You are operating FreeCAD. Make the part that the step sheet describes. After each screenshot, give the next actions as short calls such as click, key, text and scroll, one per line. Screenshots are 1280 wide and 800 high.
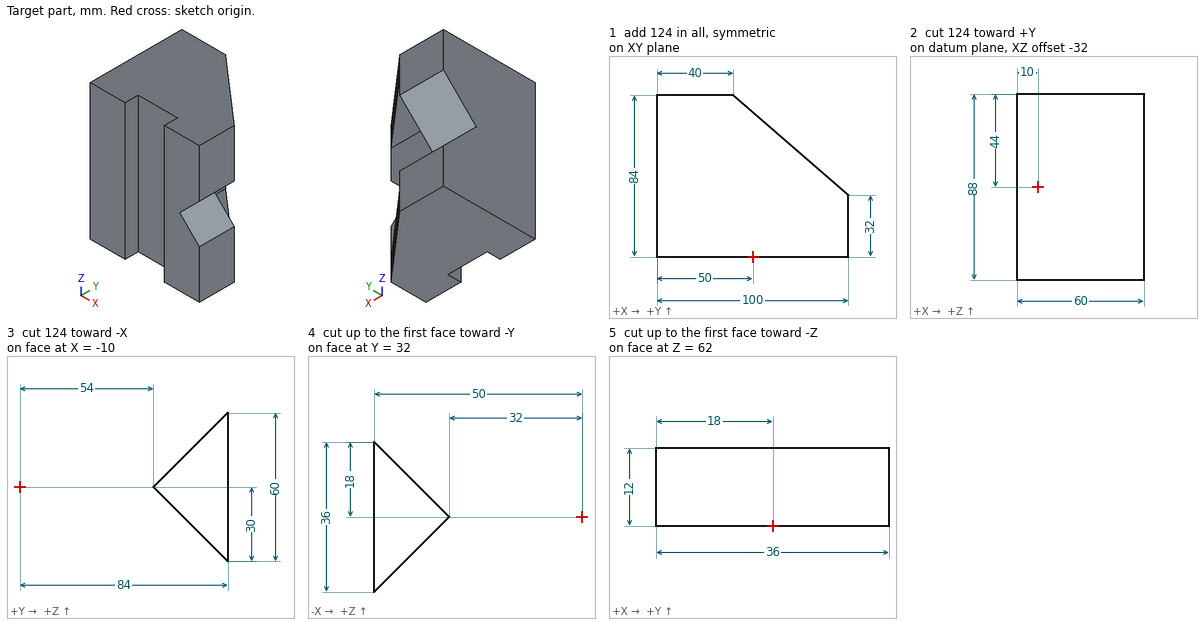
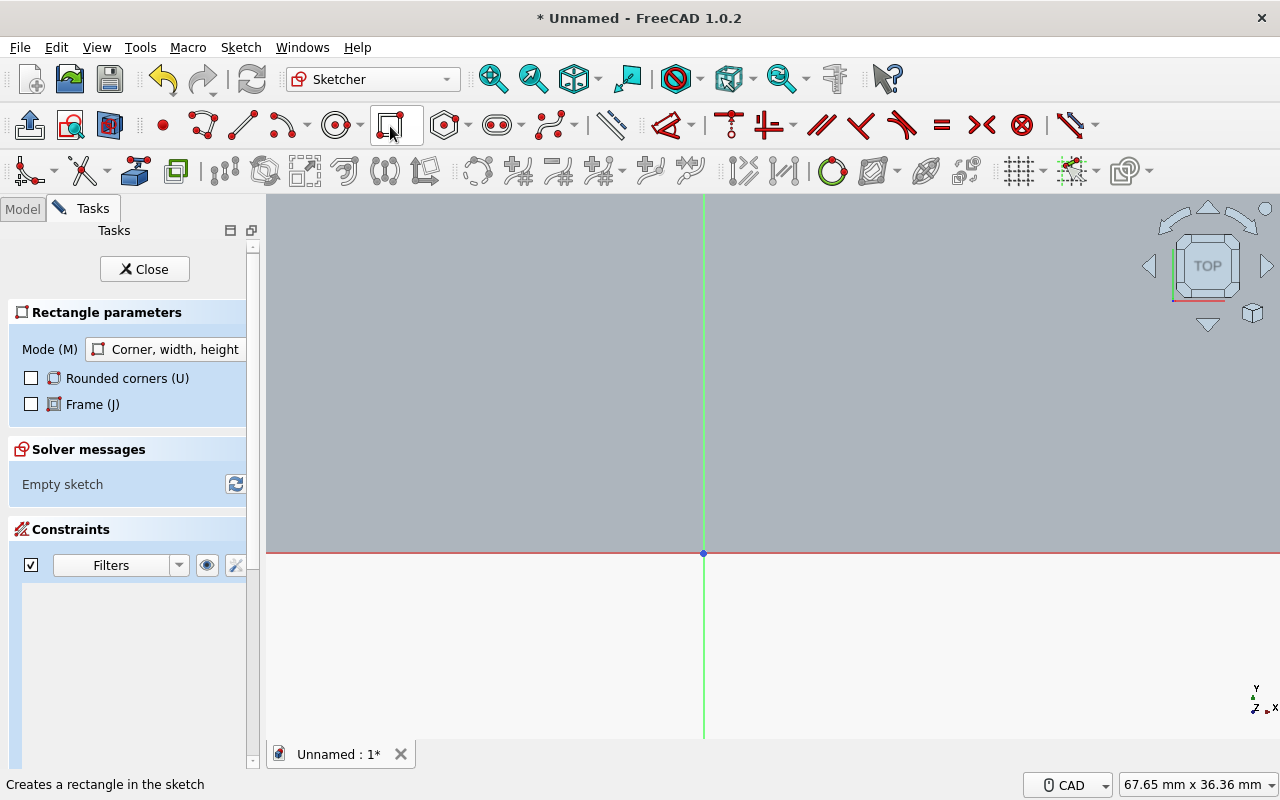
click(434, 374)
click(974, 553)
key(Escape)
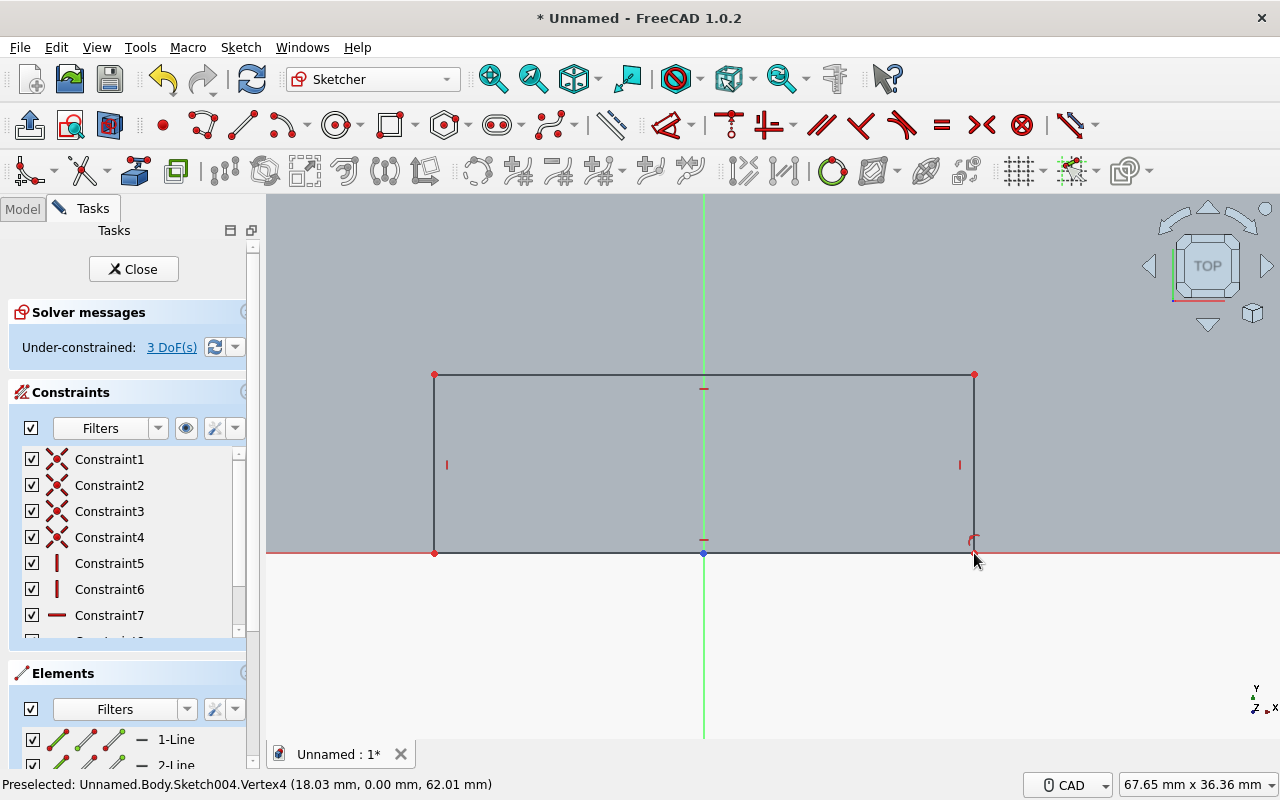
click(666, 126)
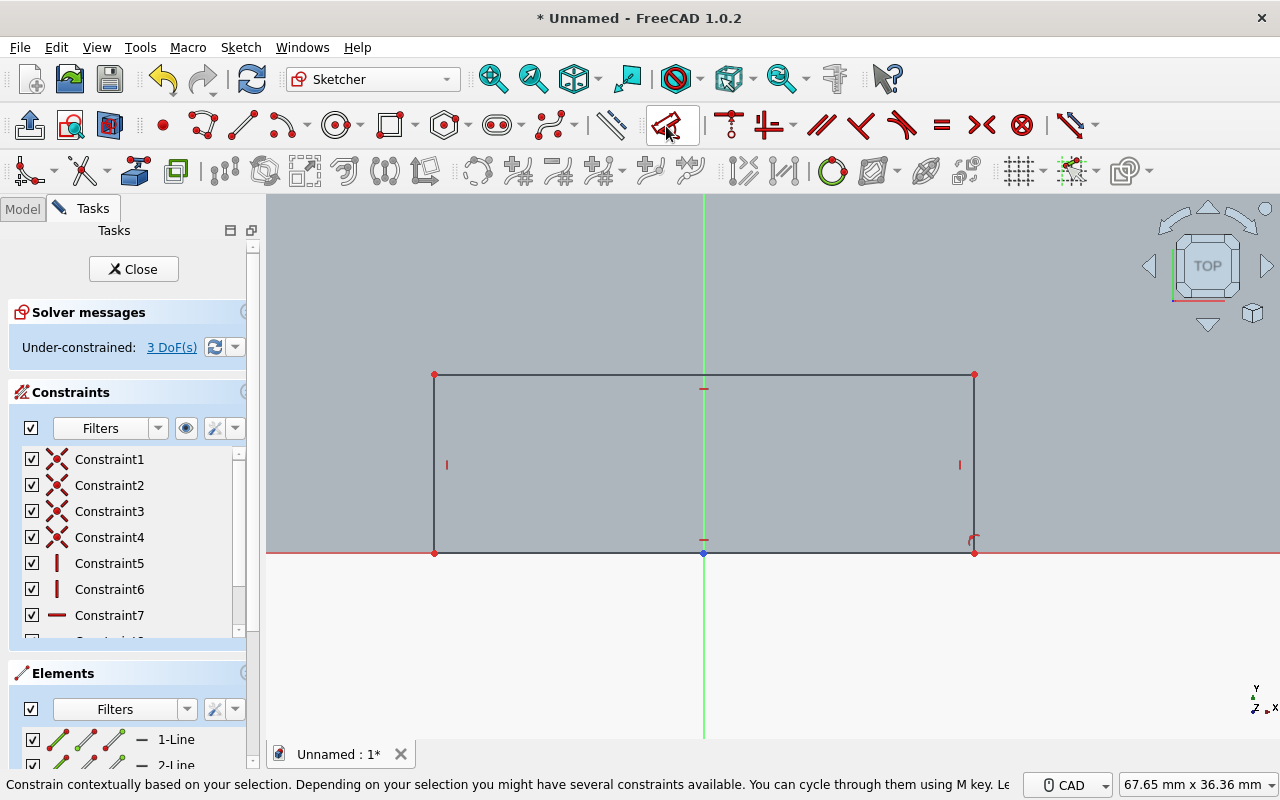
click(434, 429)
click(400, 464)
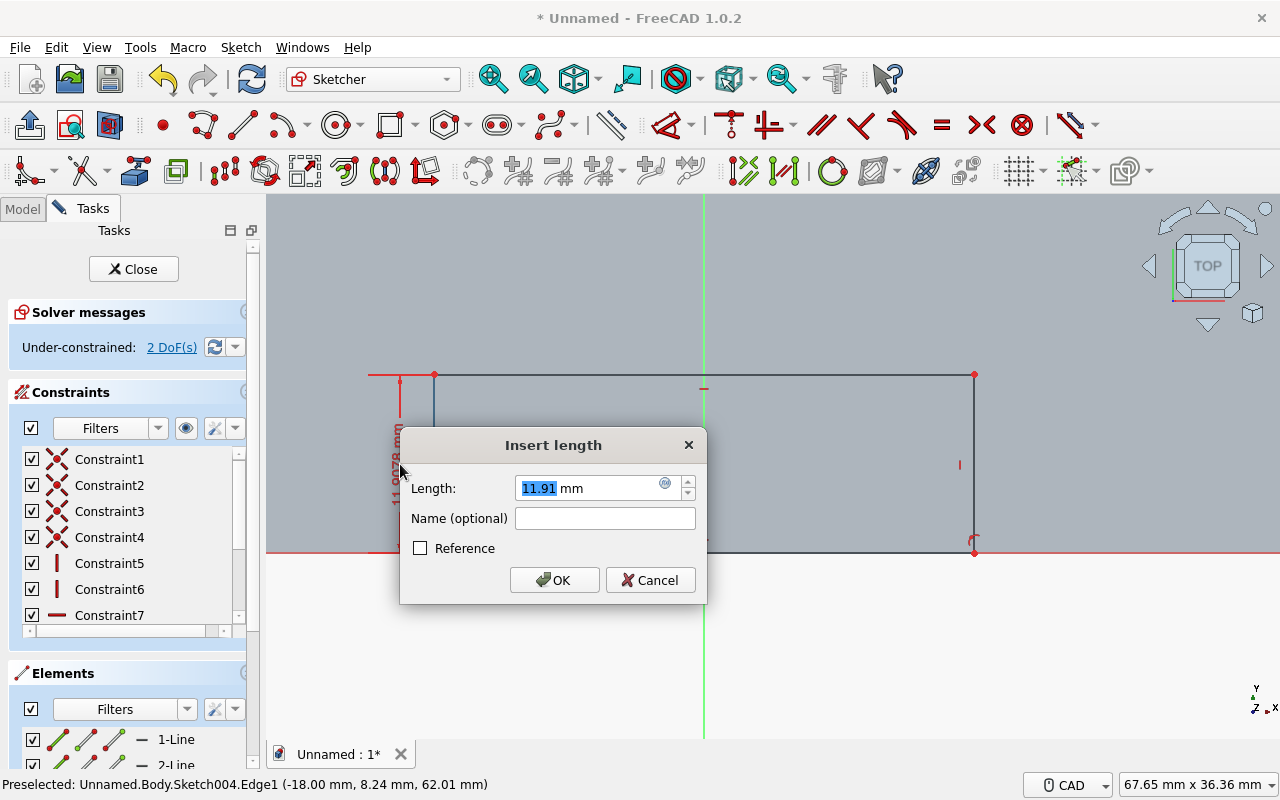
text(12)
key(Return)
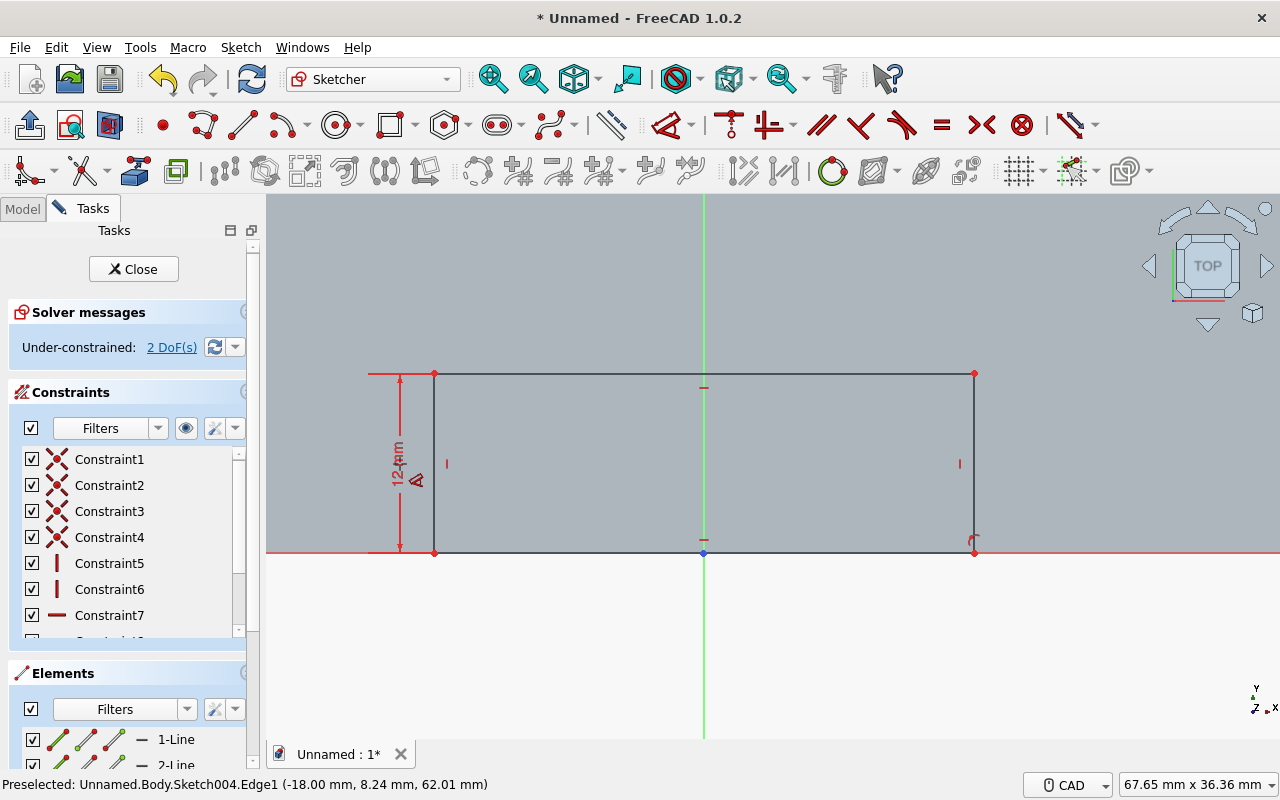
click(596, 553)
click(580, 587)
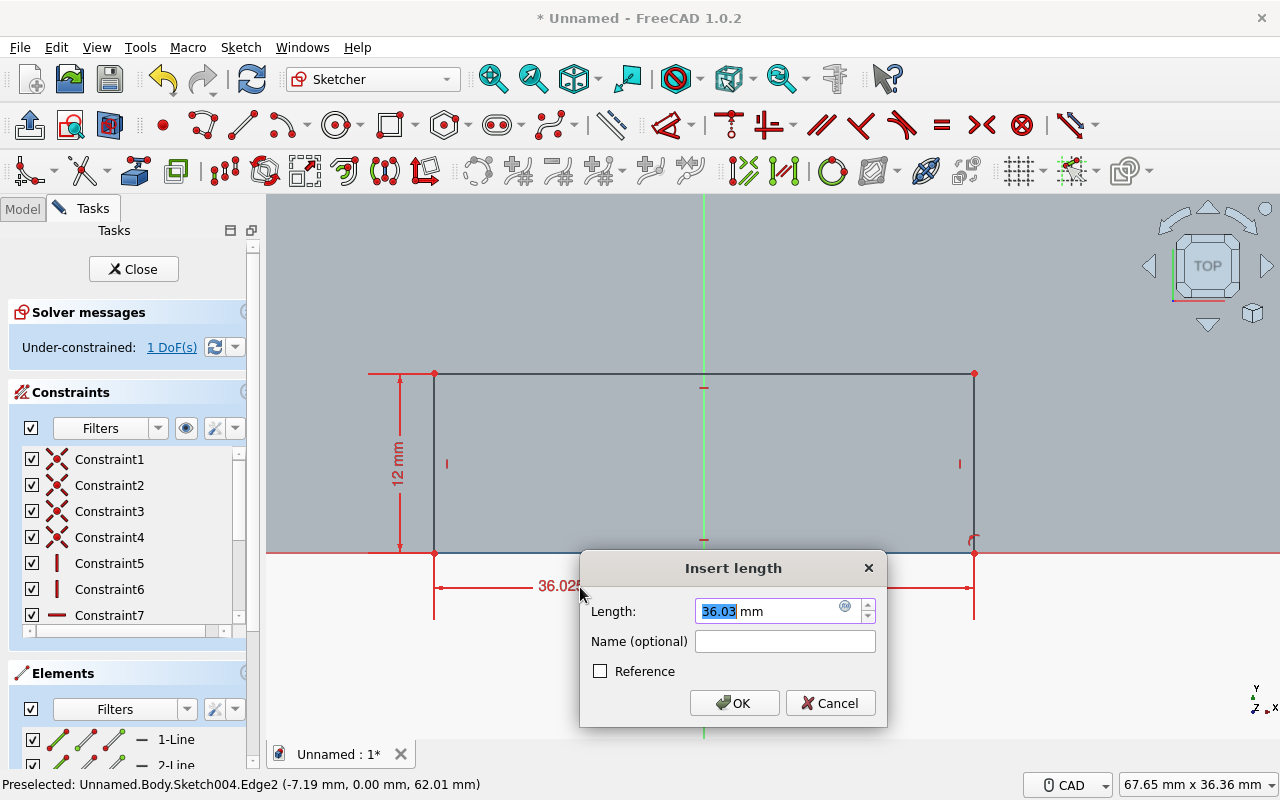
text(36)
key(Return)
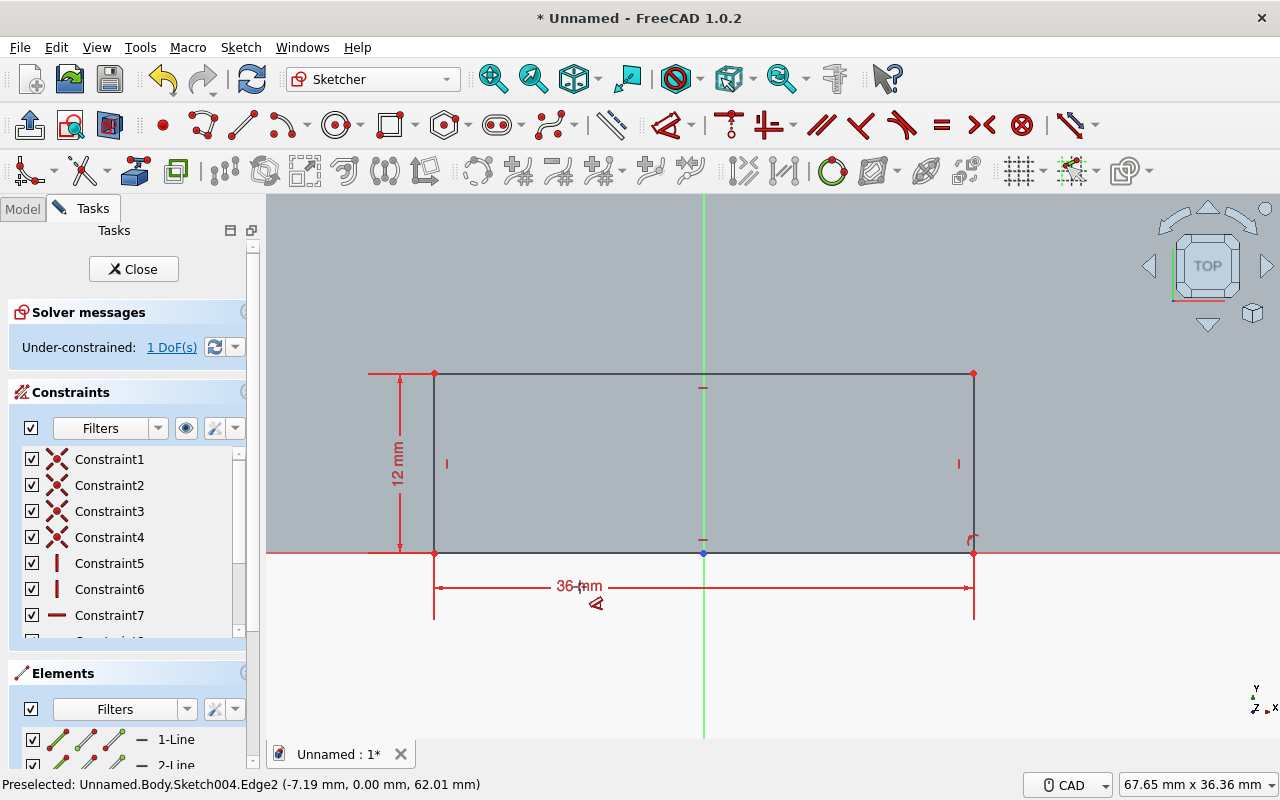
click(434, 374)
click(507, 587)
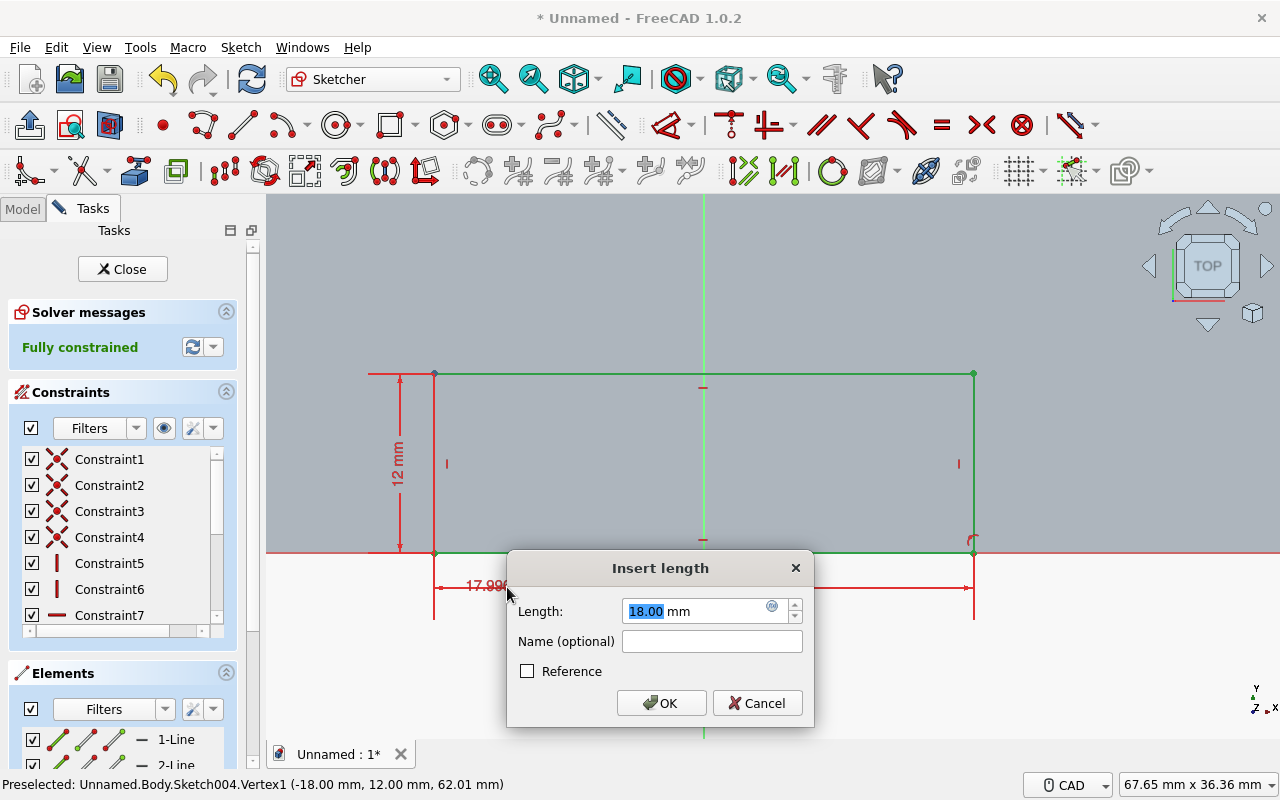
text(18)
key(Return)
key(Escape)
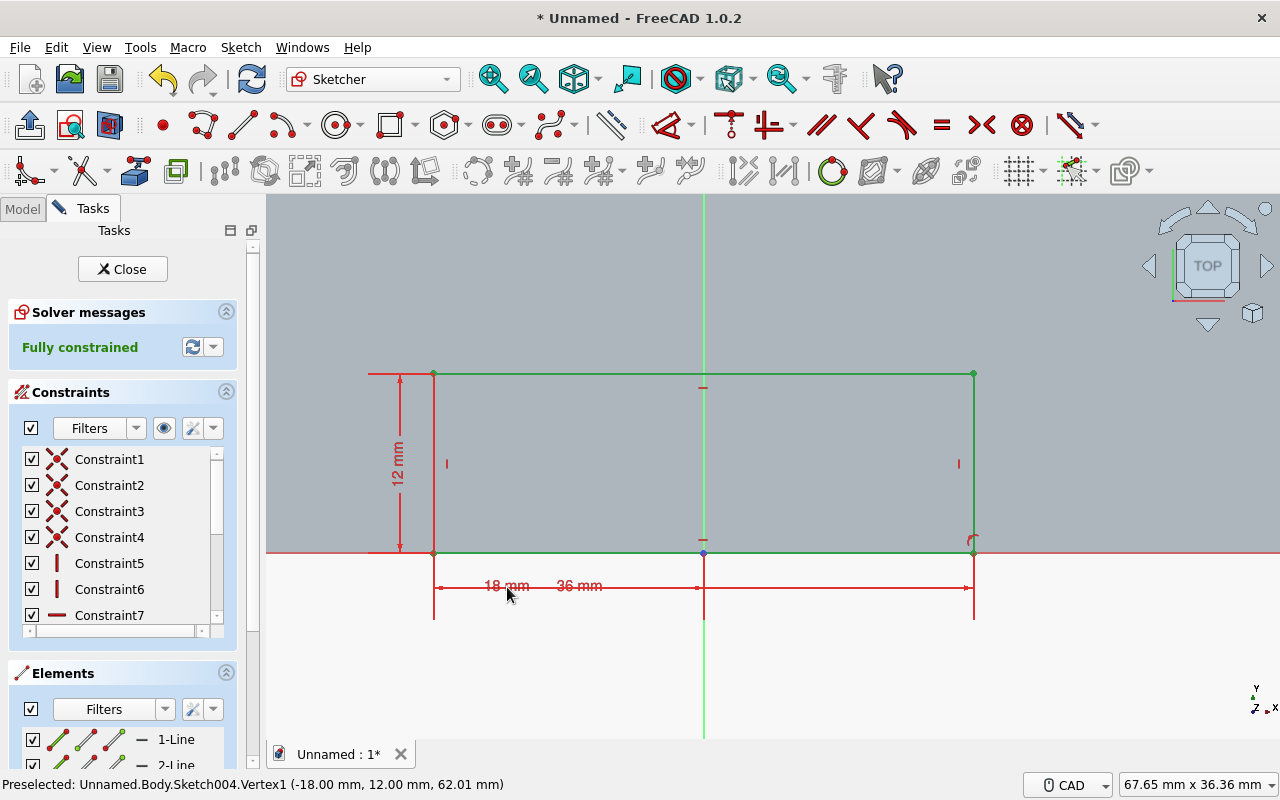
click(123, 269)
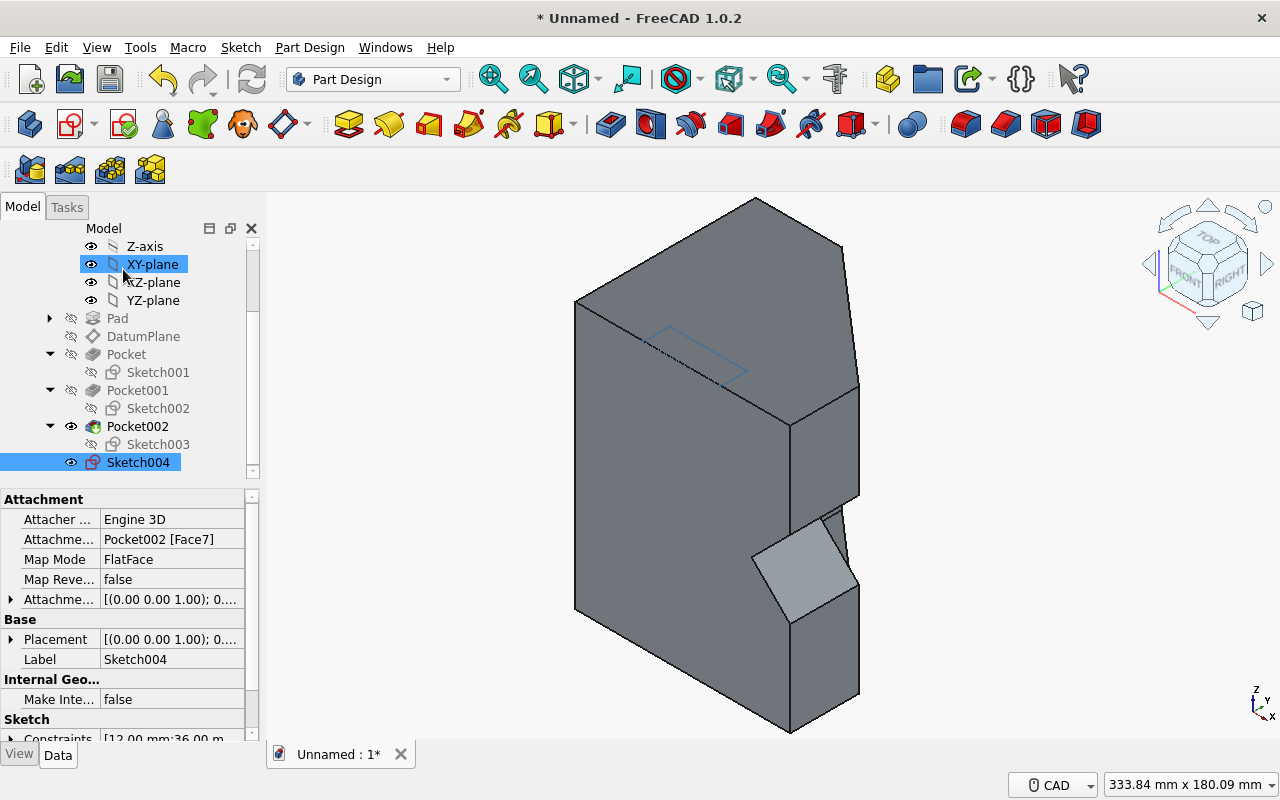
click(612, 124)